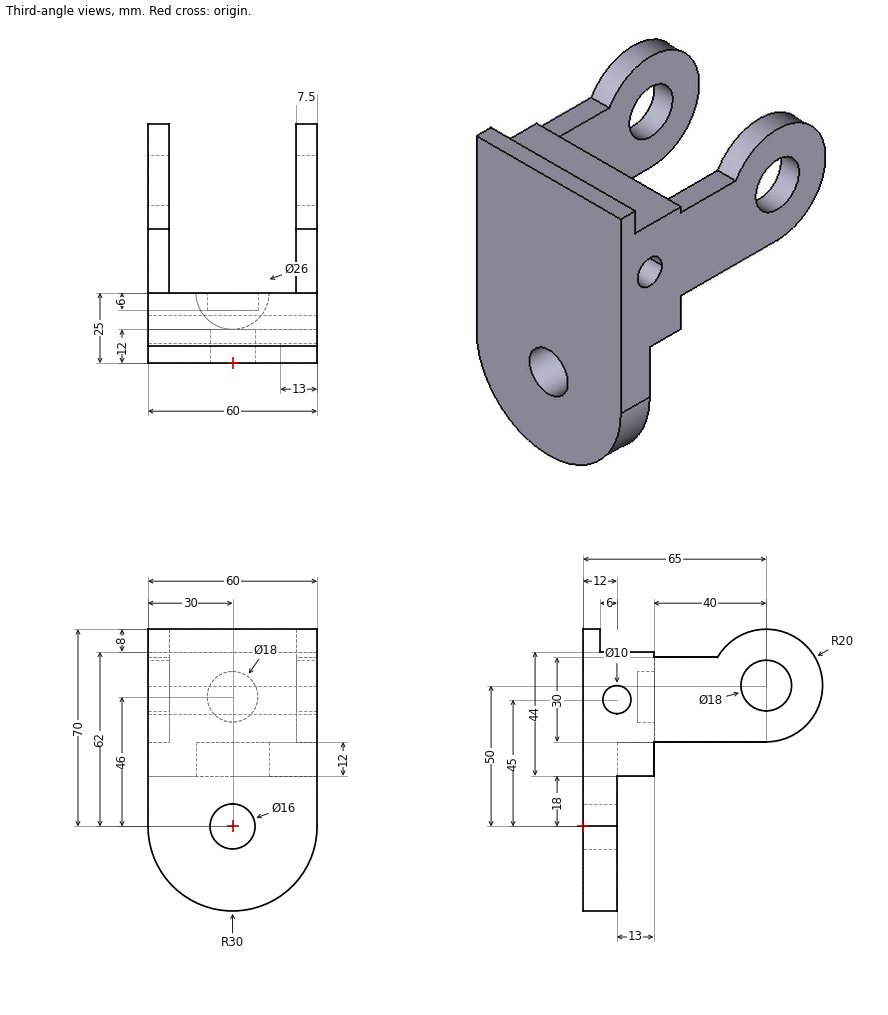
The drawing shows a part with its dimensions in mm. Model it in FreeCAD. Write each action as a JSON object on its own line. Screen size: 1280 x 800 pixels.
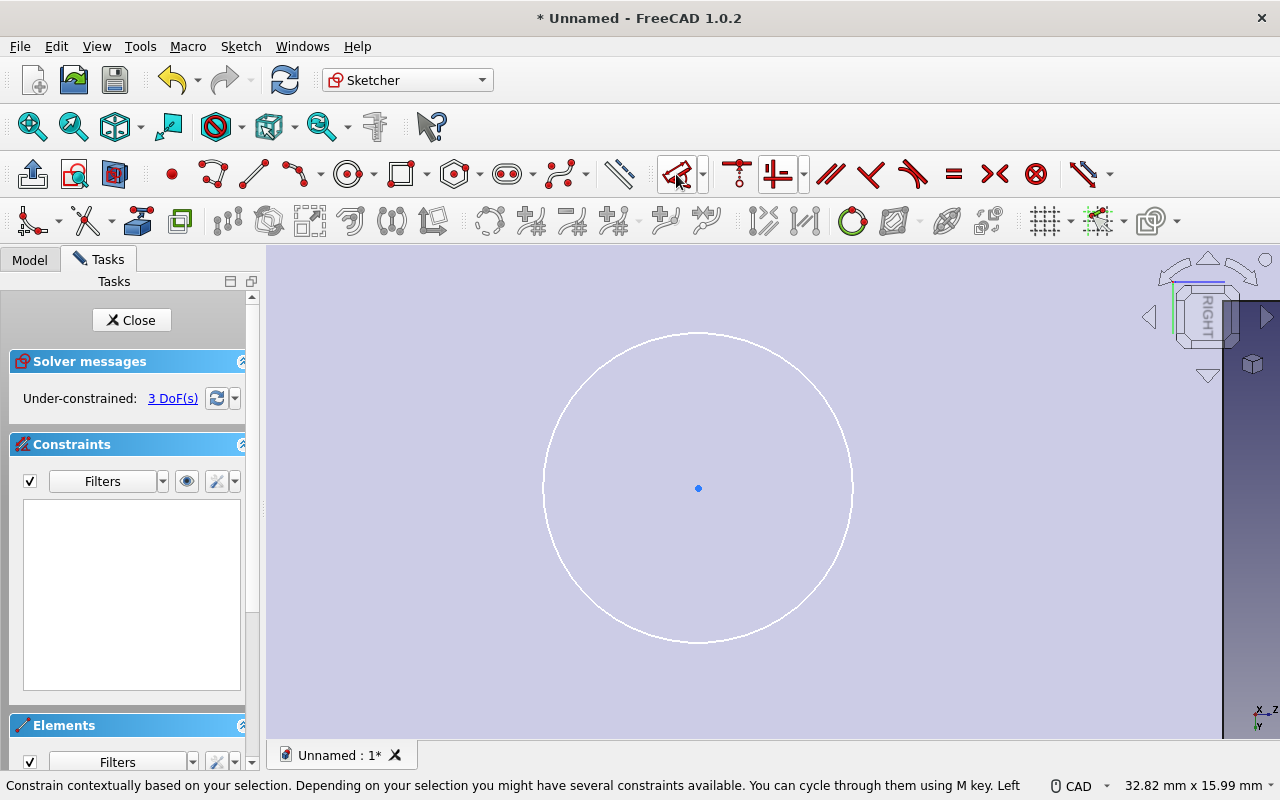
{"action": "left_click", "coordinate": [807, 378]}
{"action": "left_click", "coordinate": [830, 355]}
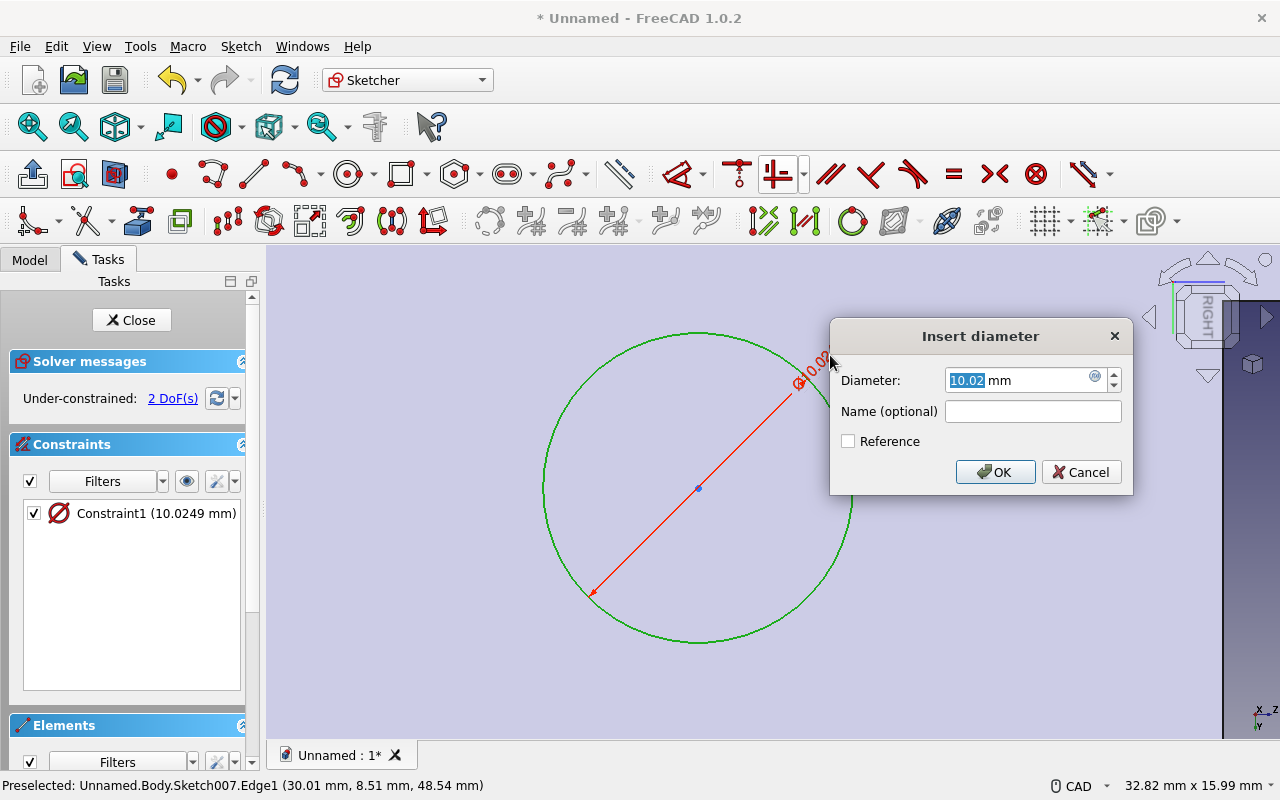
{"action": "type", "text": "10"}
{"action": "key", "text": "Return"}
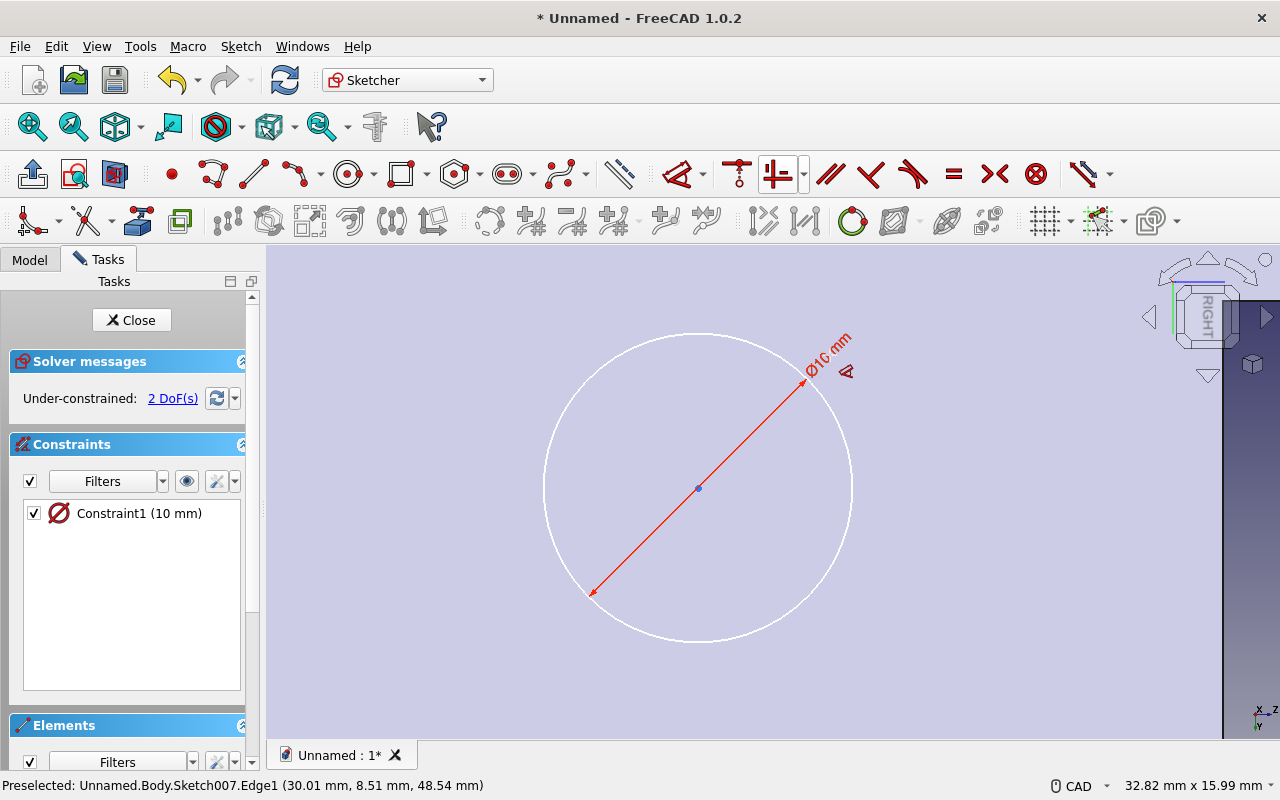
{"action": "left_click", "coordinate": [698, 488]}
{"action": "left_click", "coordinate": [496, 522]}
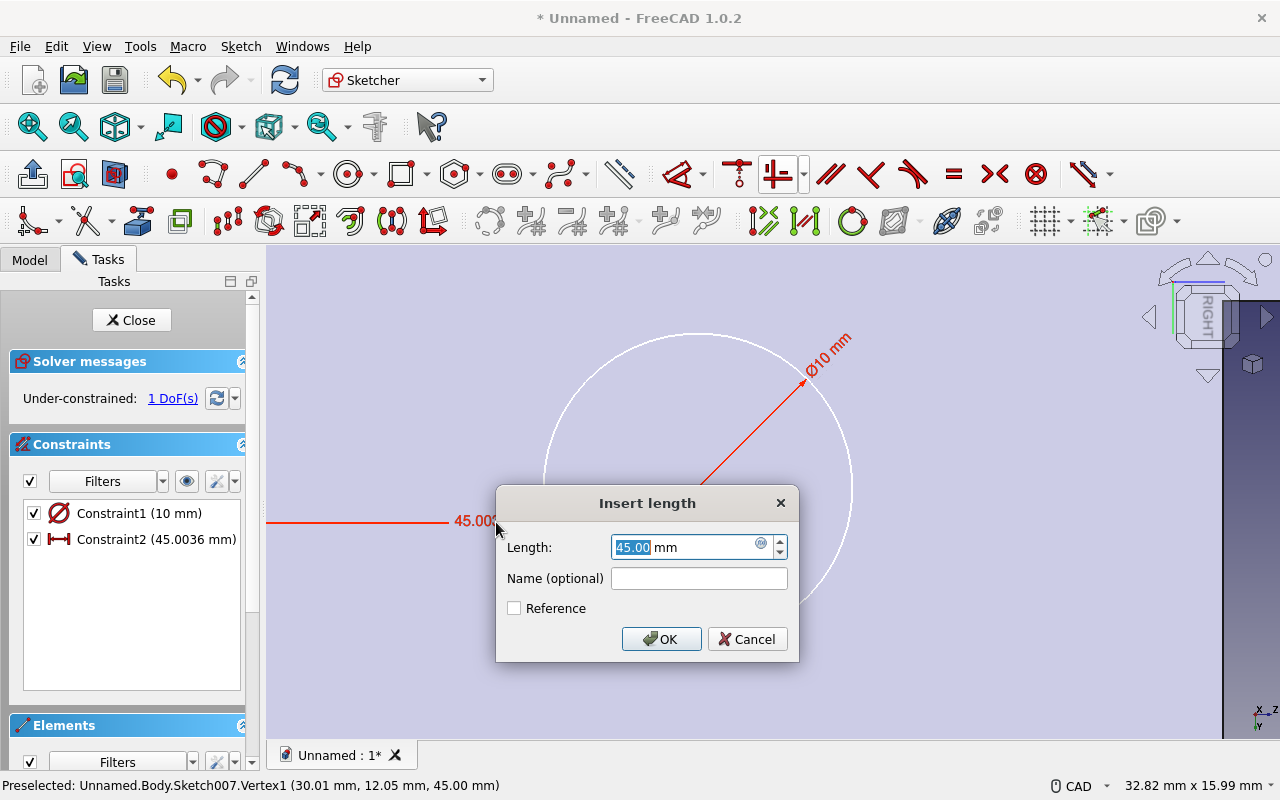
{"action": "type", "text": "45"}
{"action": "key", "text": "Return"}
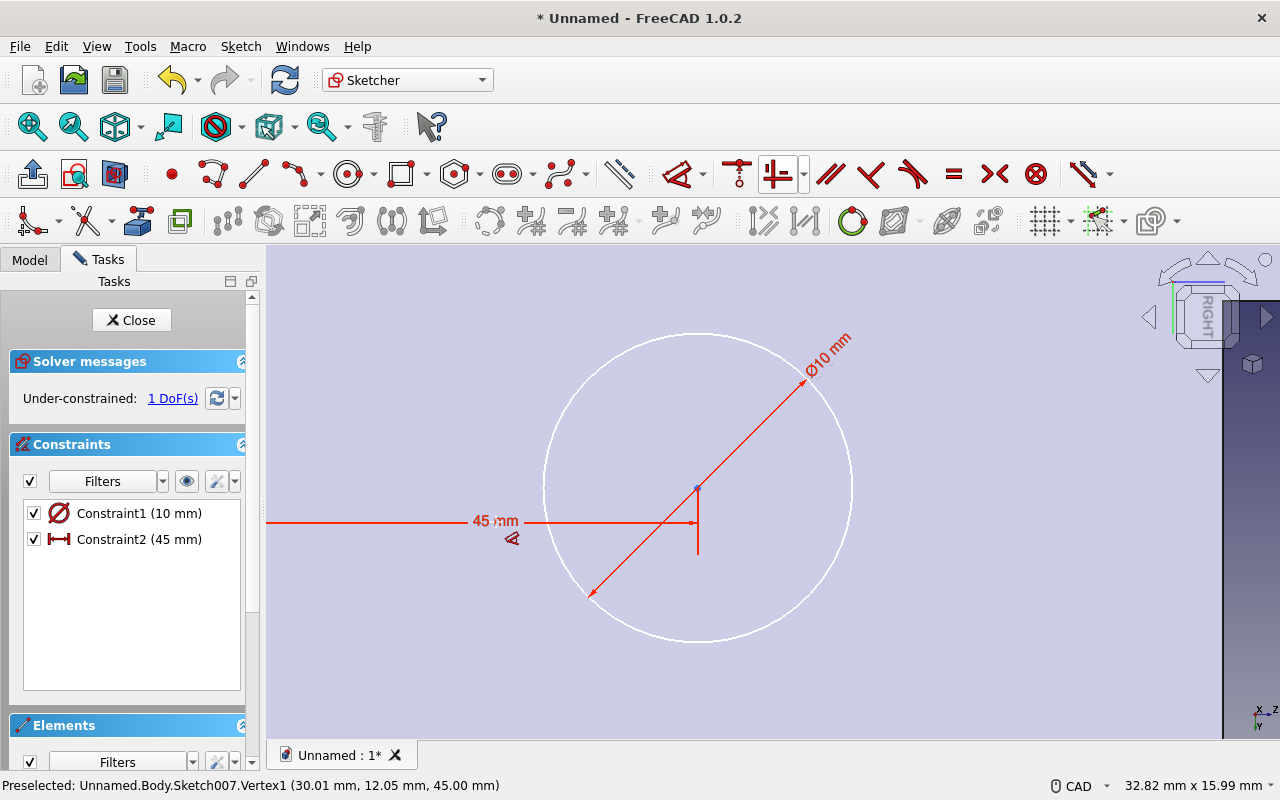
{"action": "left_click", "coordinate": [698, 488]}
{"action": "left_click", "coordinate": [732, 381]}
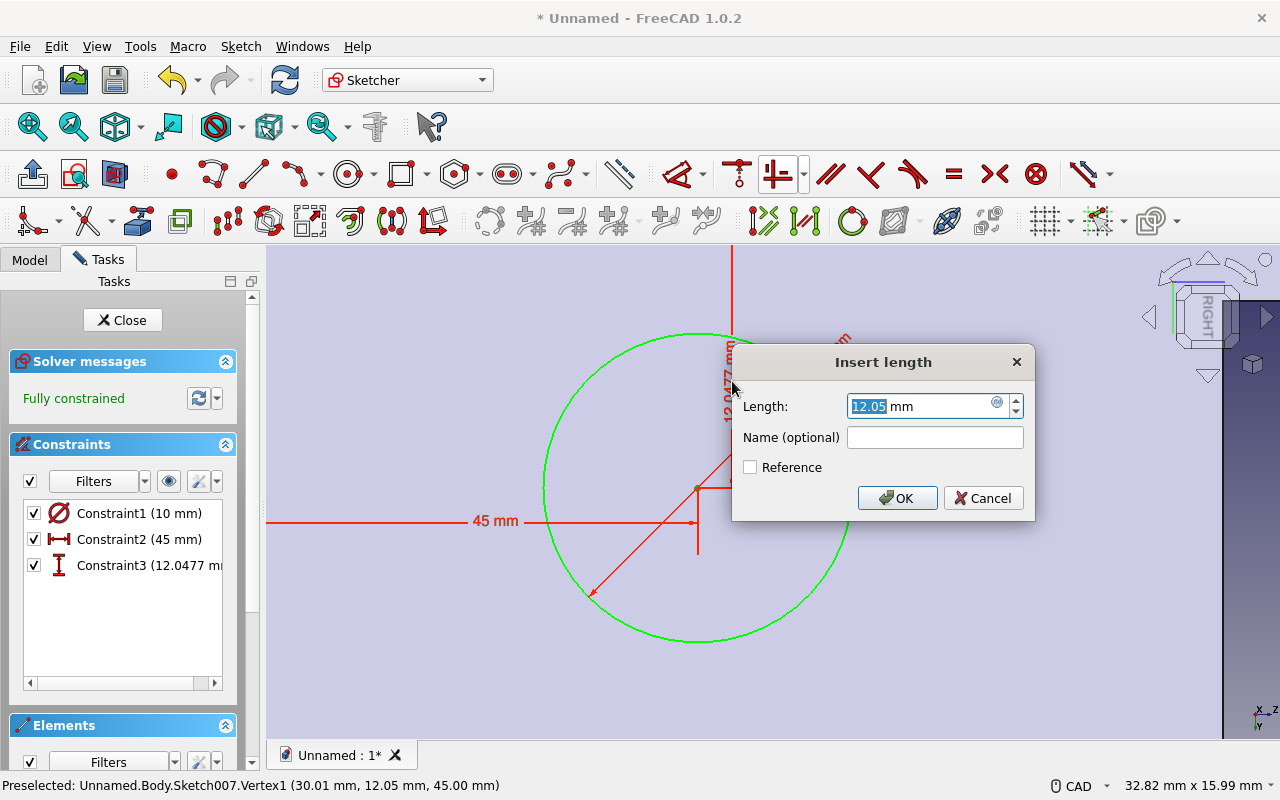
{"action": "type", "text": "12"}
{"action": "key", "text": "Return"}
{"action": "key", "text": "Escape"}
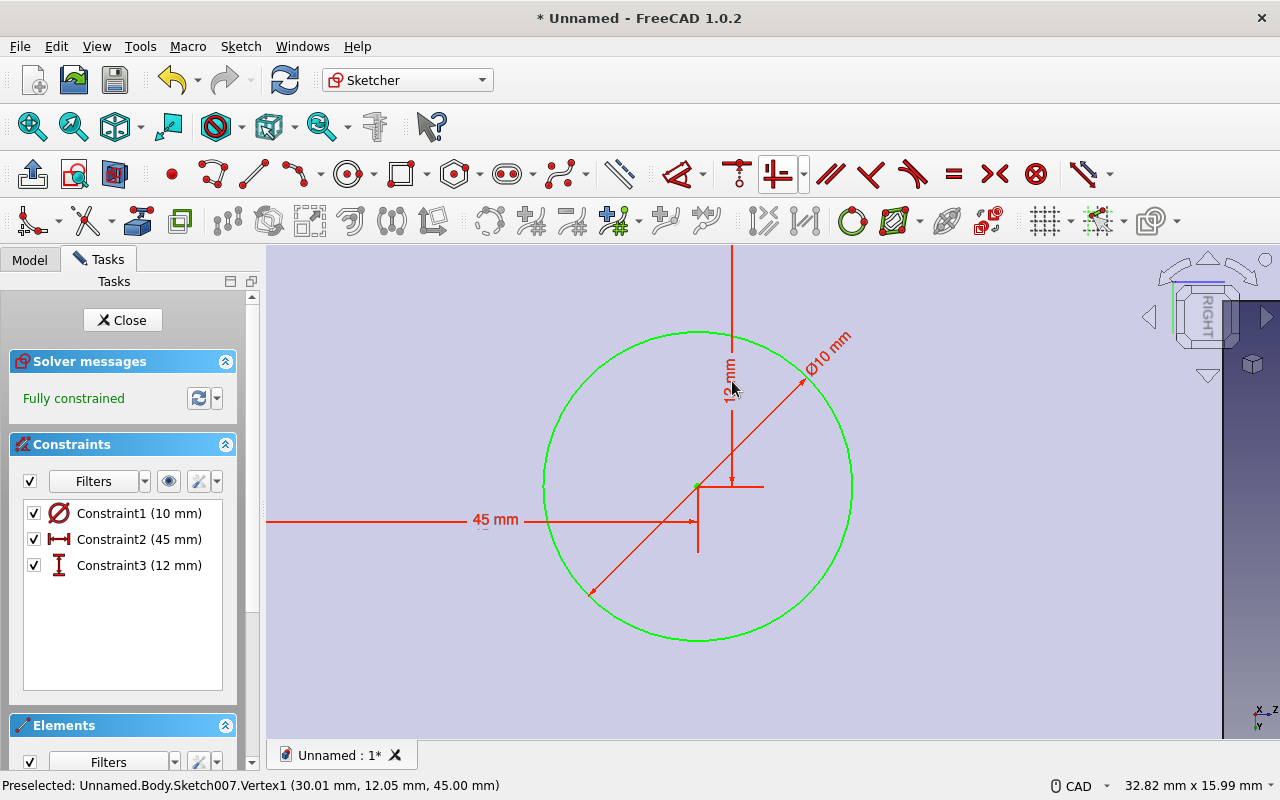
{"action": "left_click", "coordinate": [123, 320]}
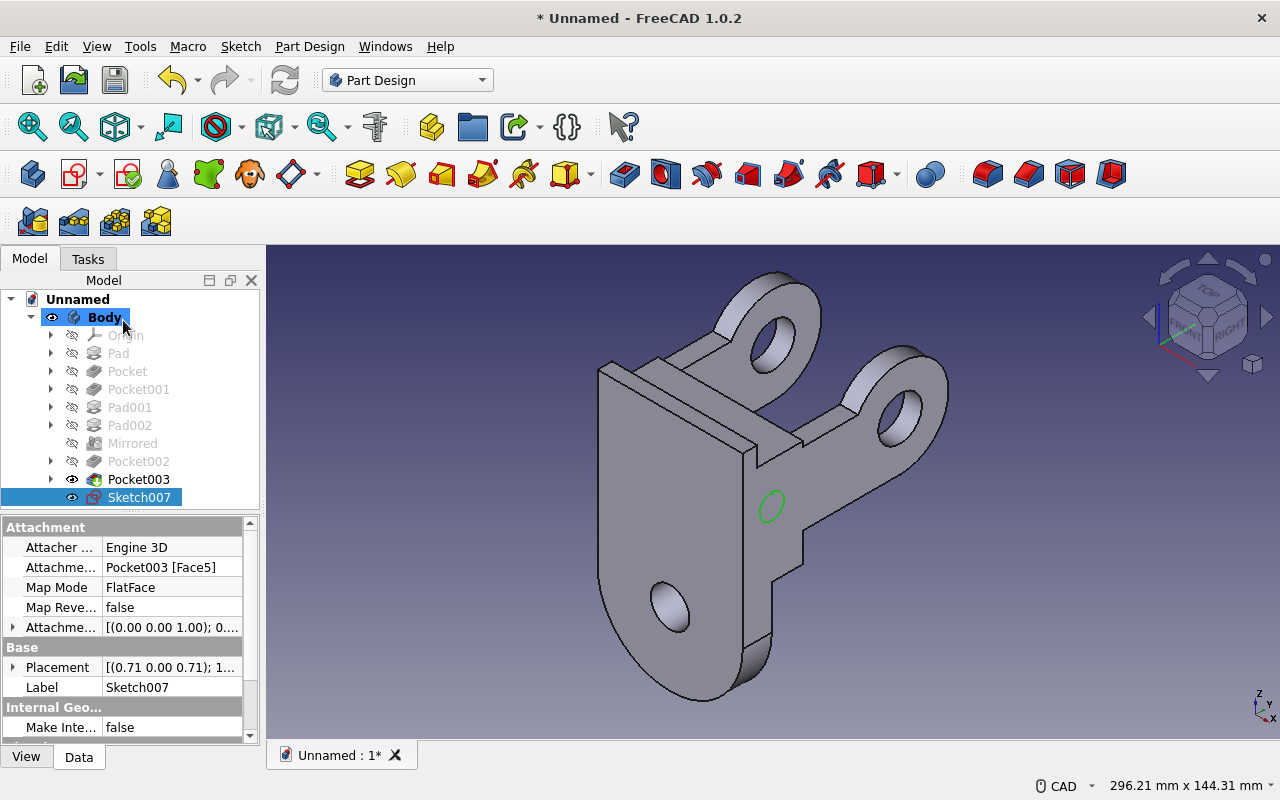
{"action": "left_click", "coordinate": [625, 174]}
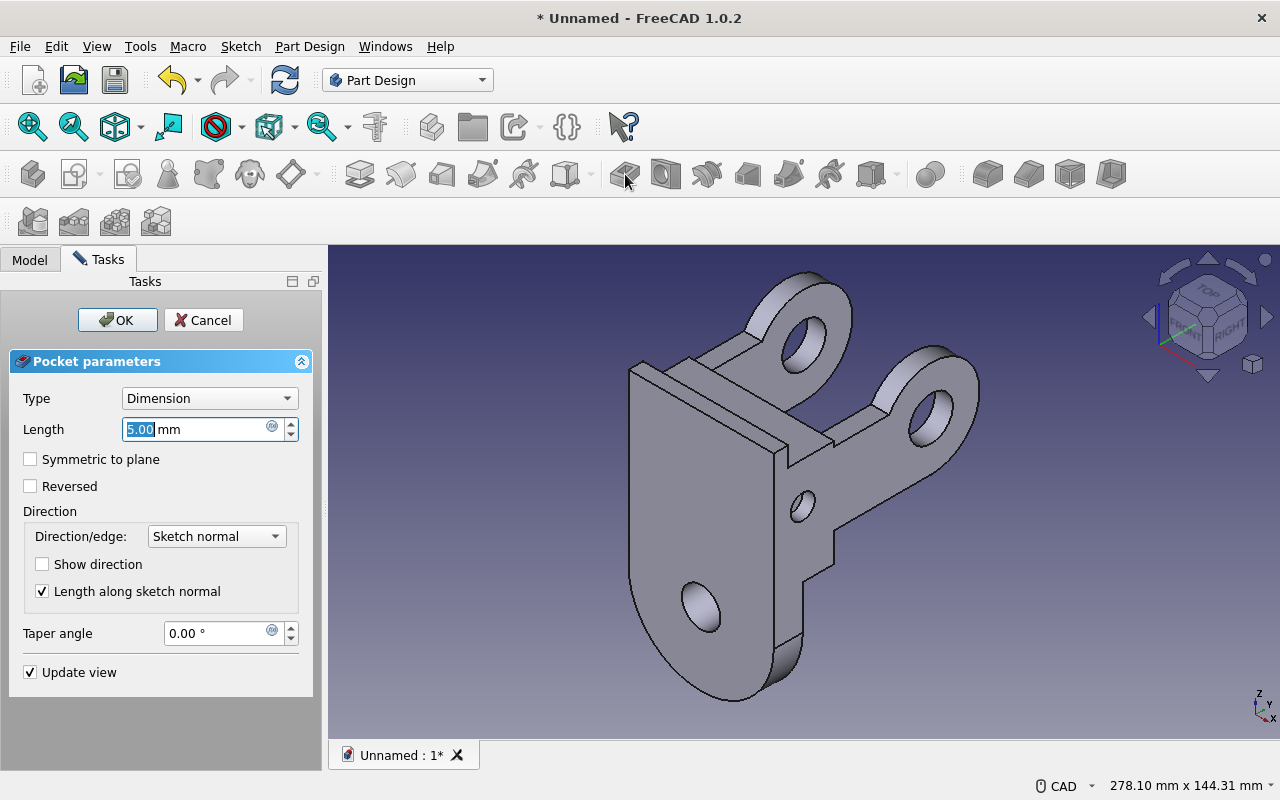
{"action": "type", "text": "13"}
{"action": "key", "text": "Tab"}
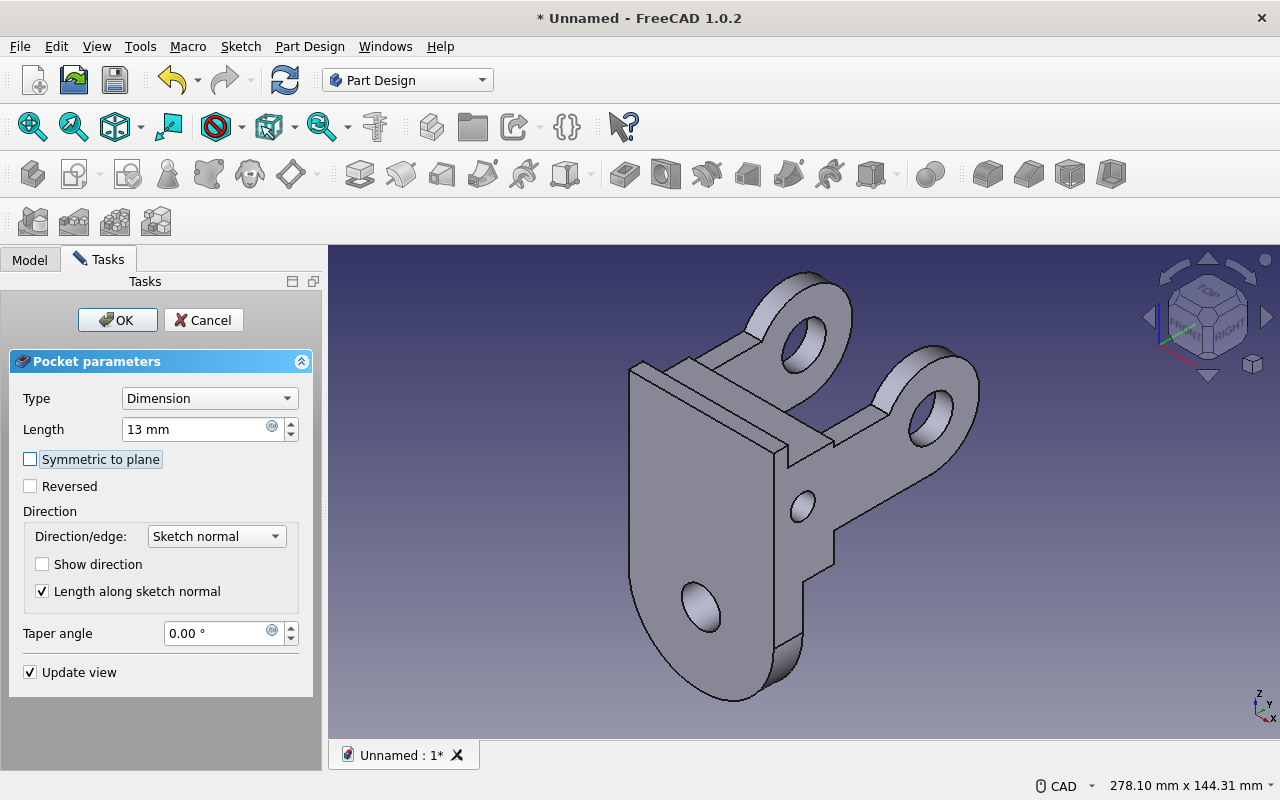
{"action": "left_click", "coordinate": [118, 320]}